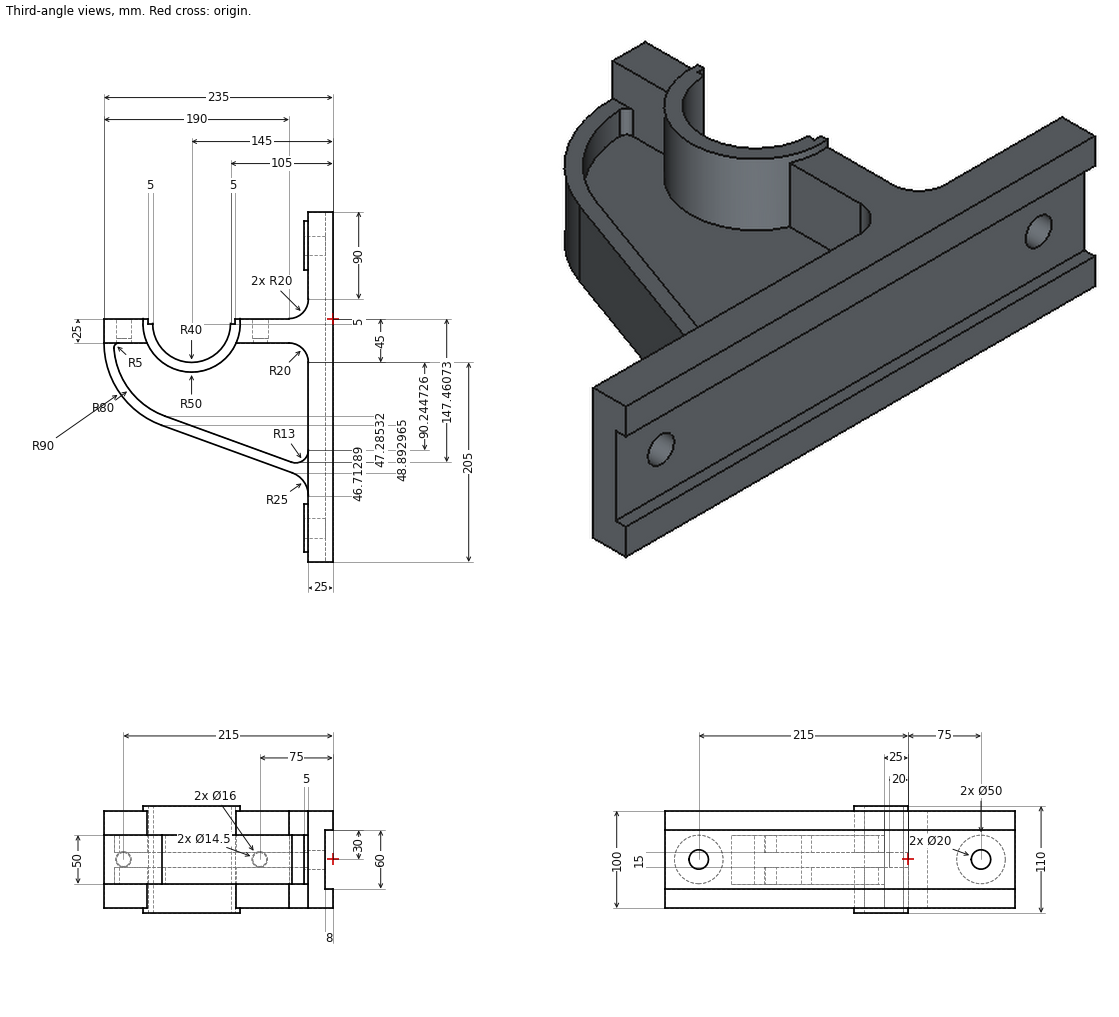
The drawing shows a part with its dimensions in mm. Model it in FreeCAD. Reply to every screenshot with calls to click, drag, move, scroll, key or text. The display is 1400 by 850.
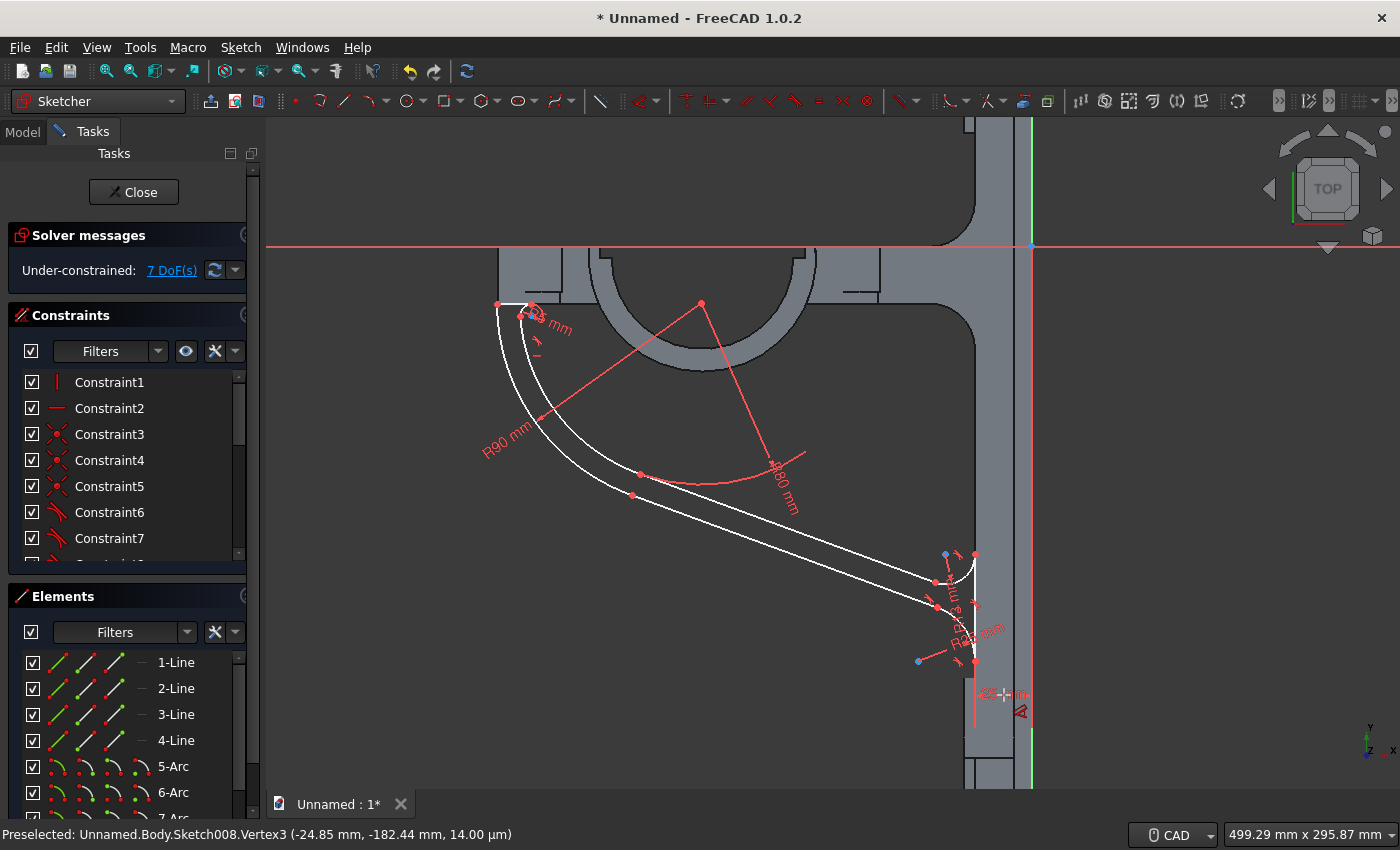
click(532, 304)
click(1066, 276)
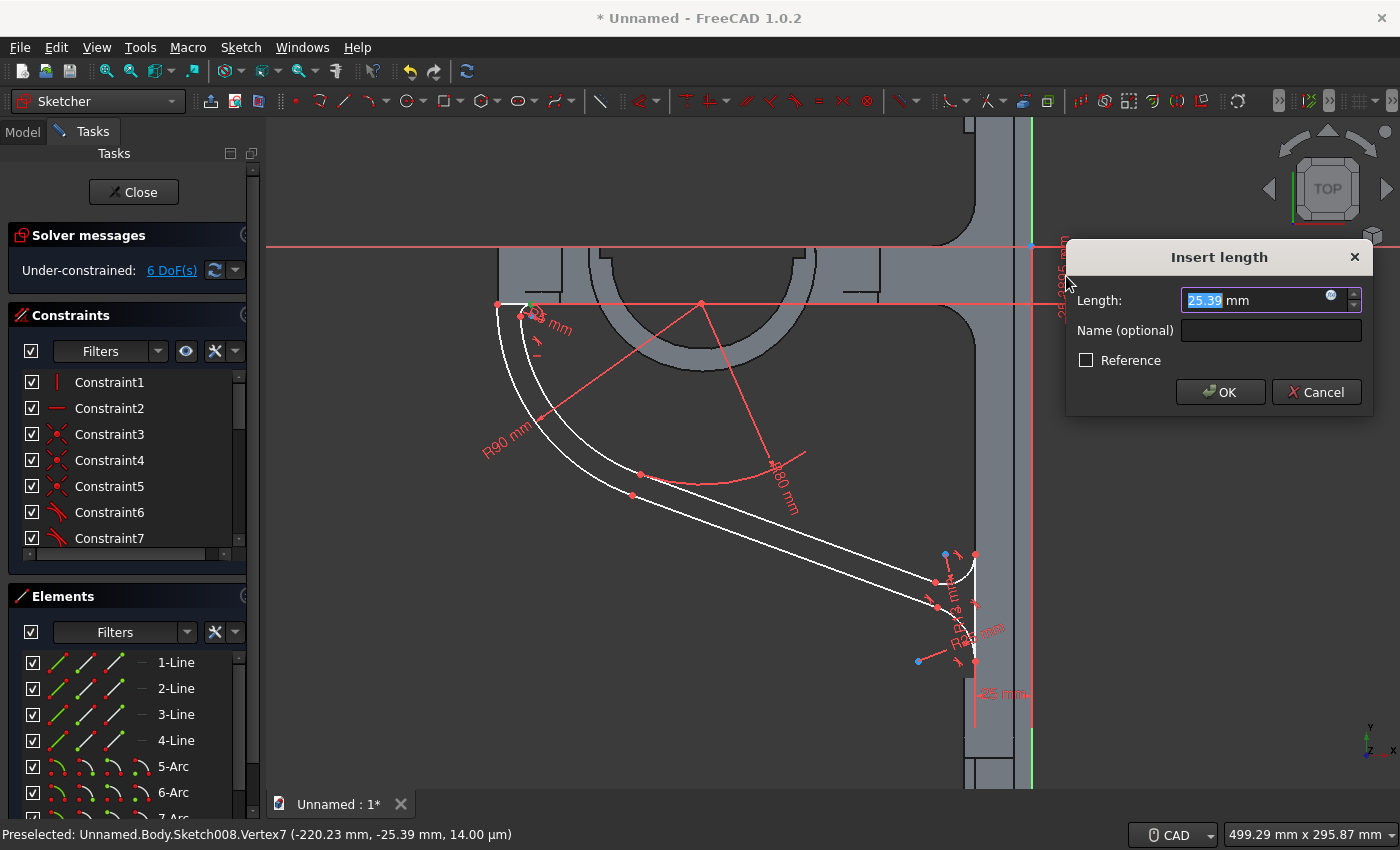
text(25)
key(Return)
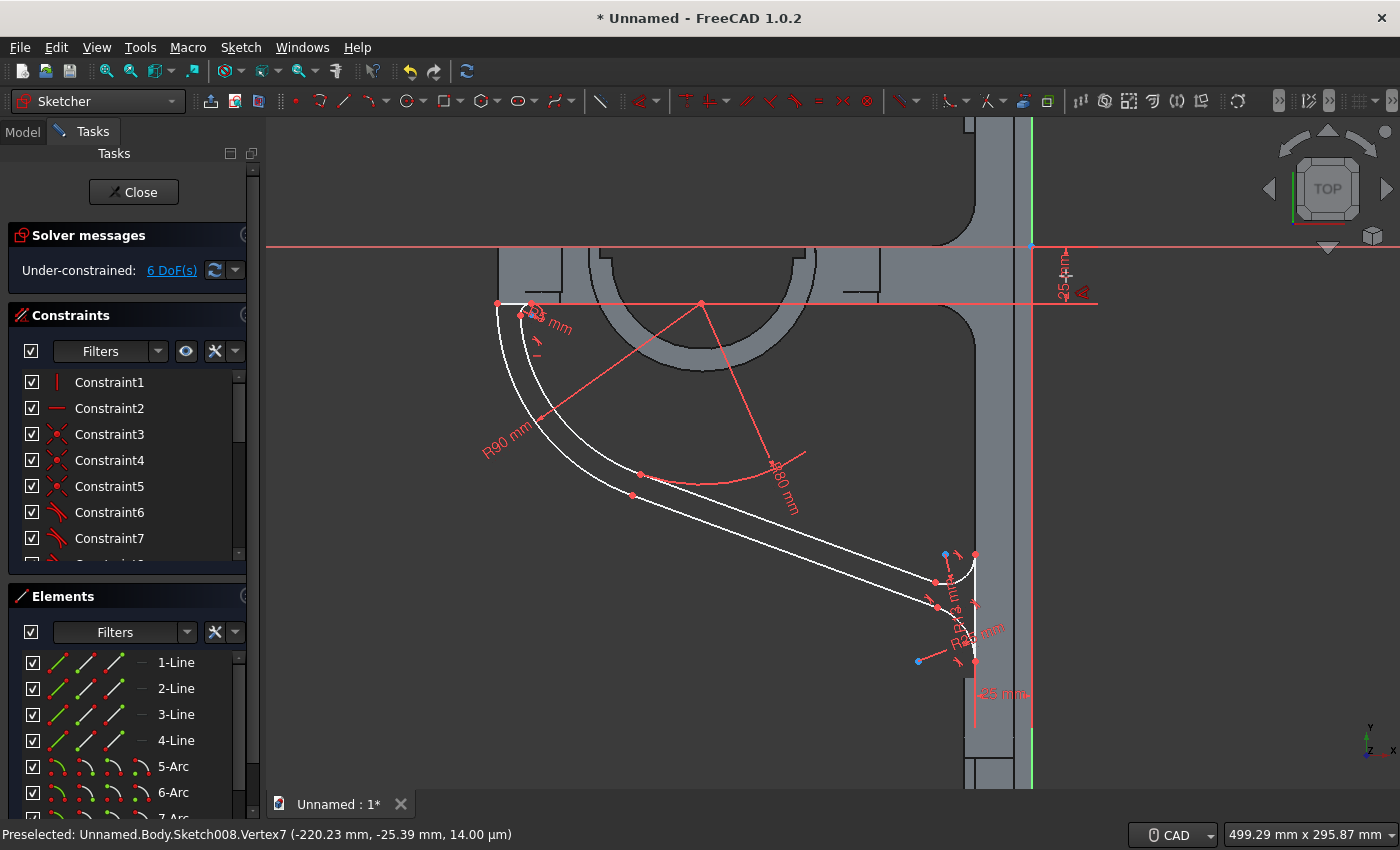
click(701, 303)
click(667, 275)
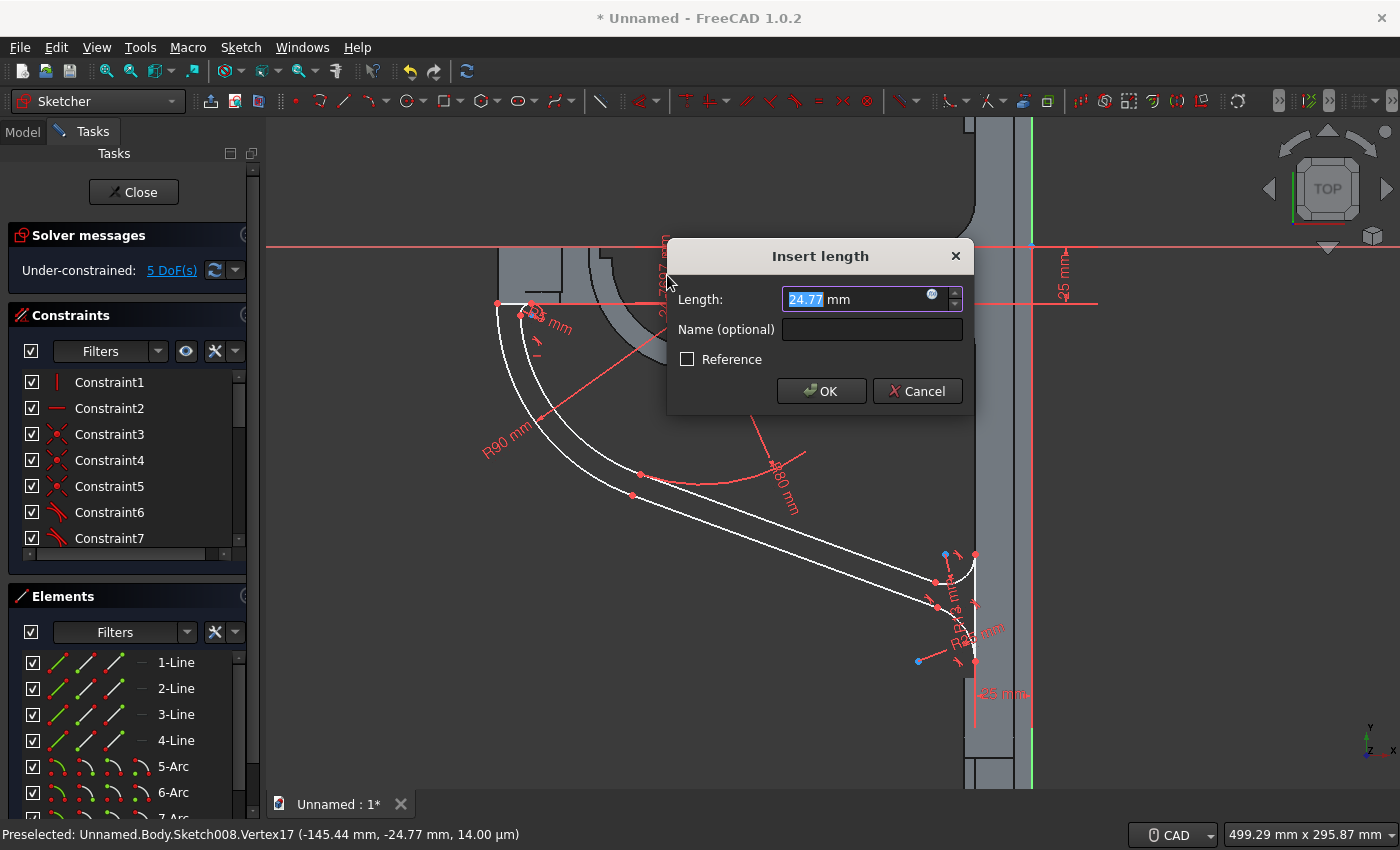
text(25)
key(Return)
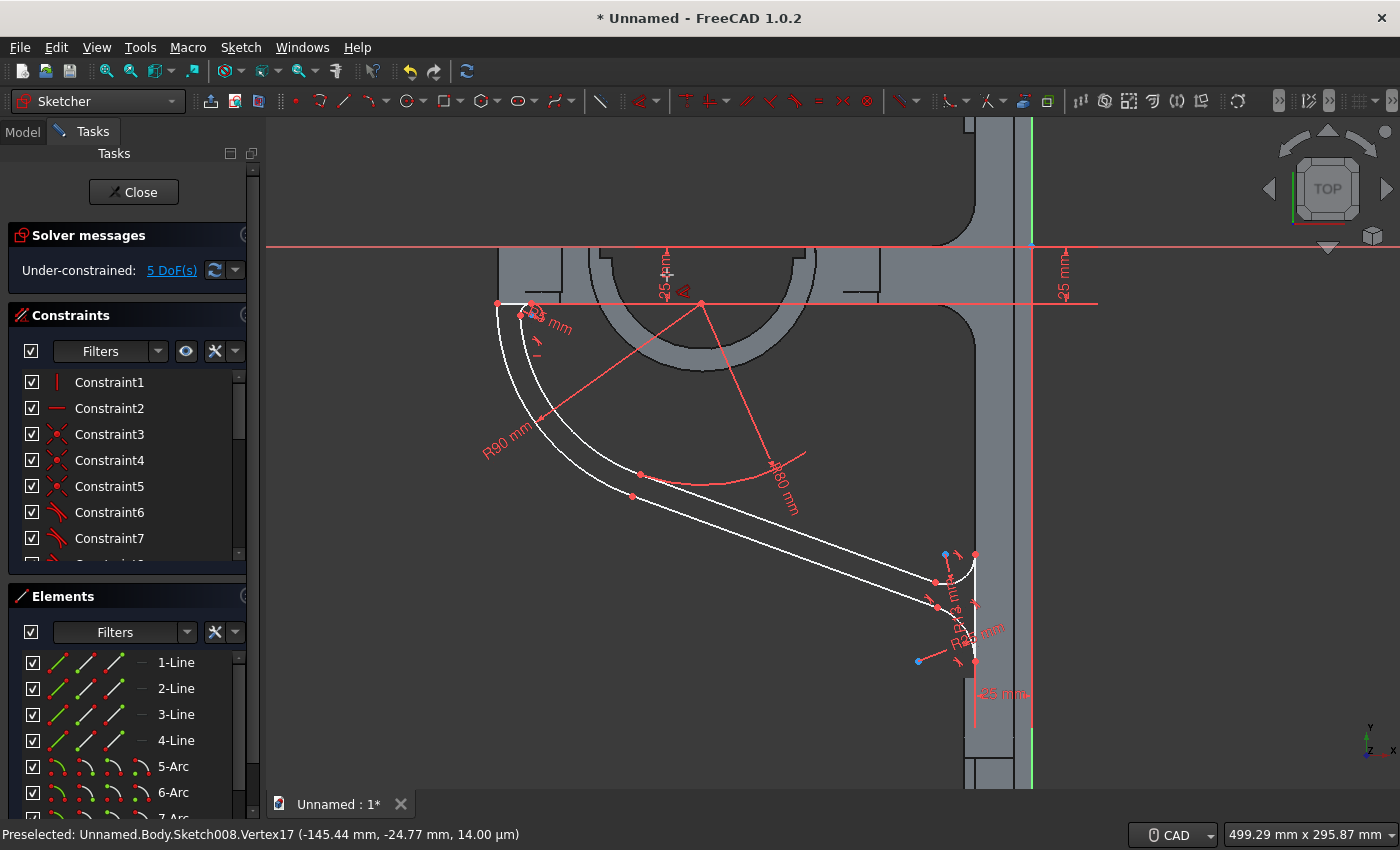
click(497, 304)
click(764, 213)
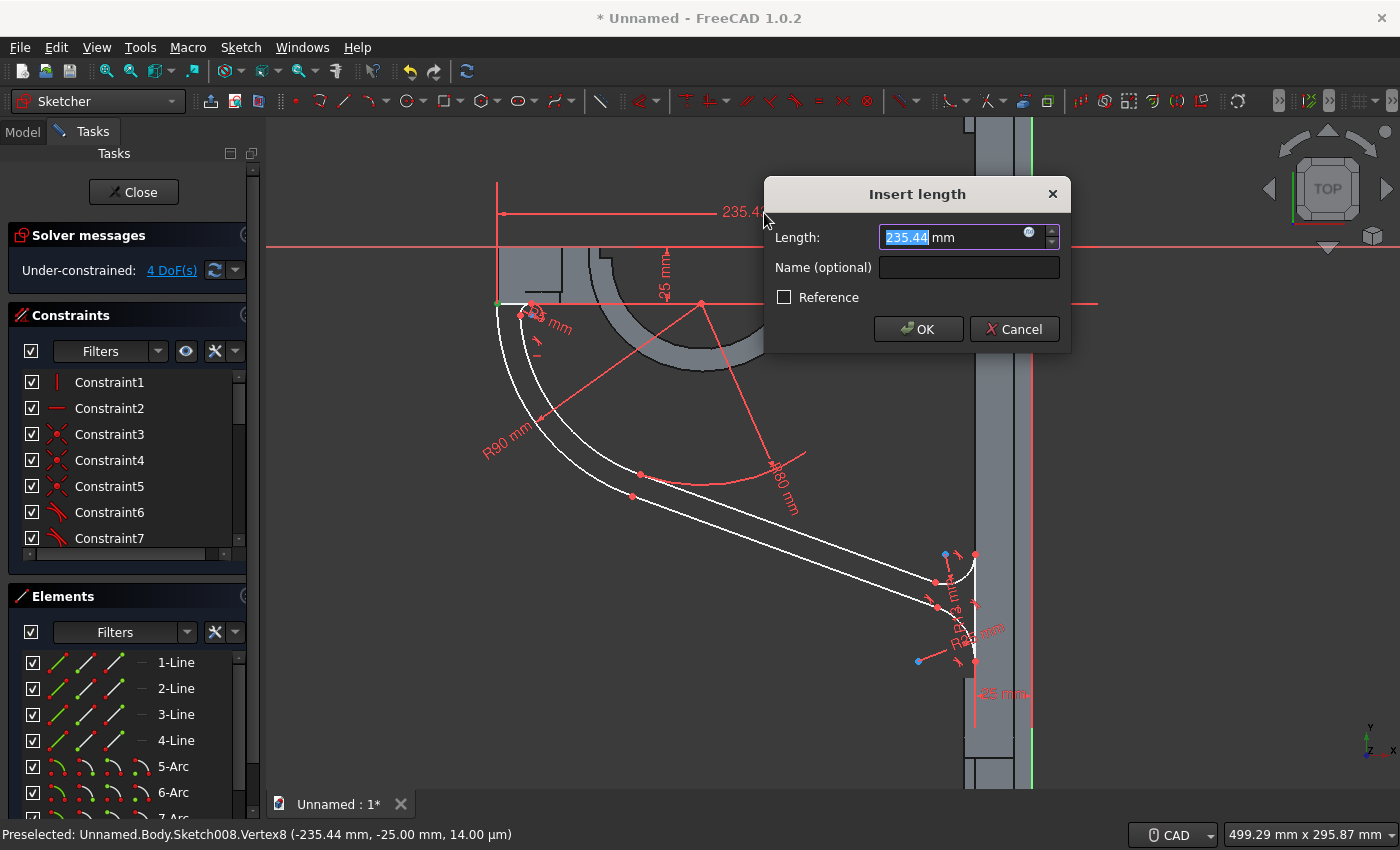
text(235)
key(Return)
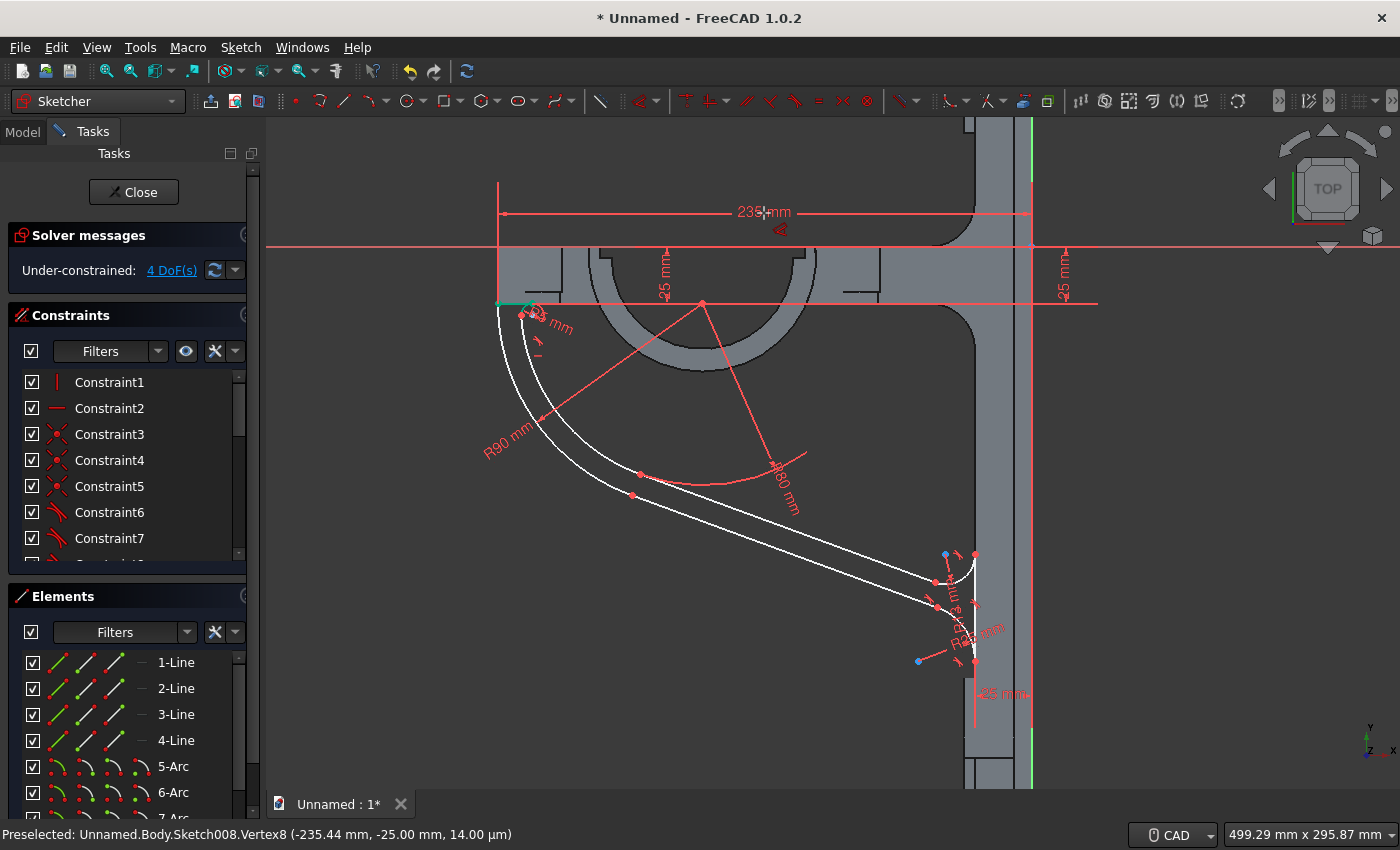
click(975, 587)
click(1009, 584)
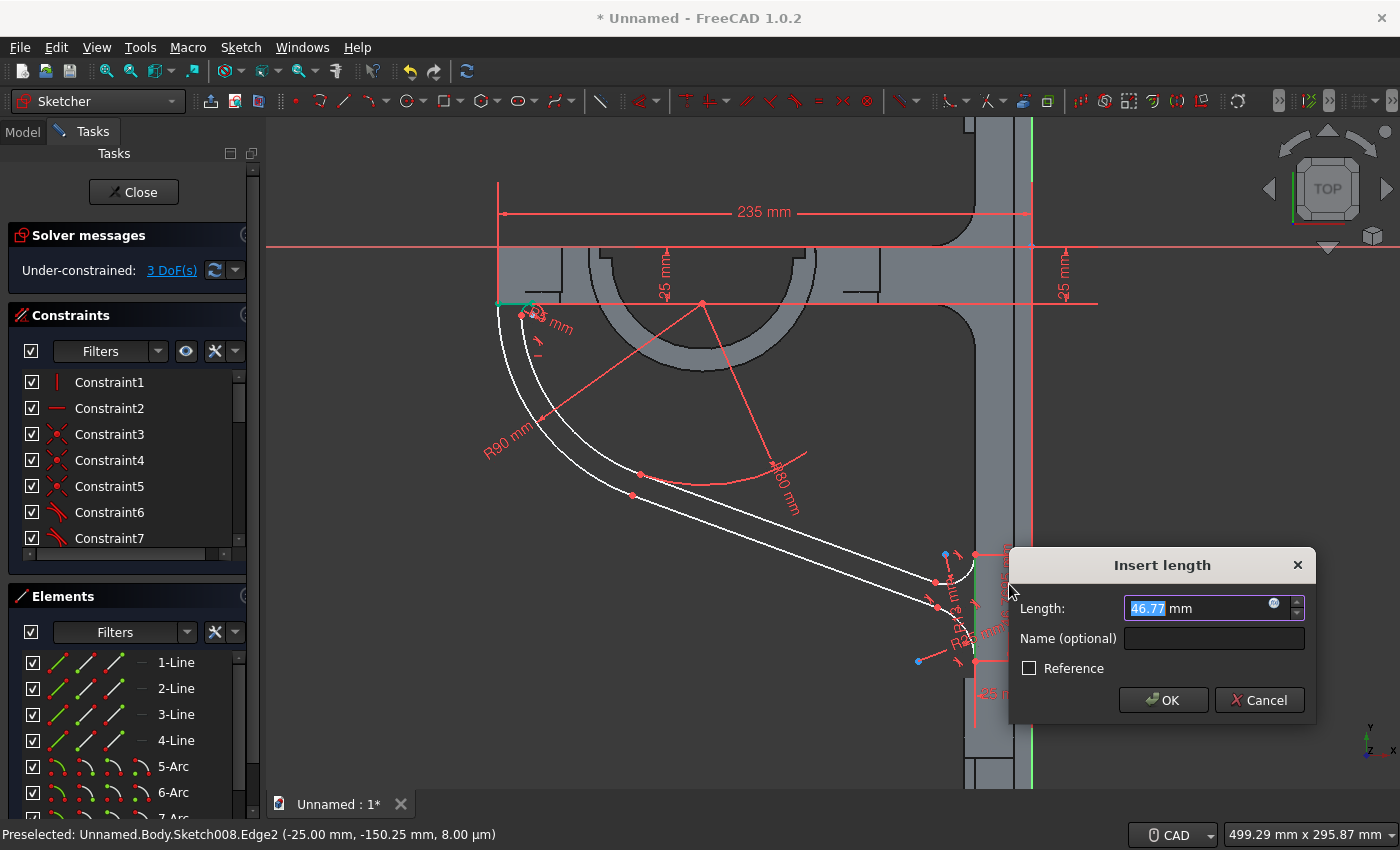
text(46.71289)
key(Return)